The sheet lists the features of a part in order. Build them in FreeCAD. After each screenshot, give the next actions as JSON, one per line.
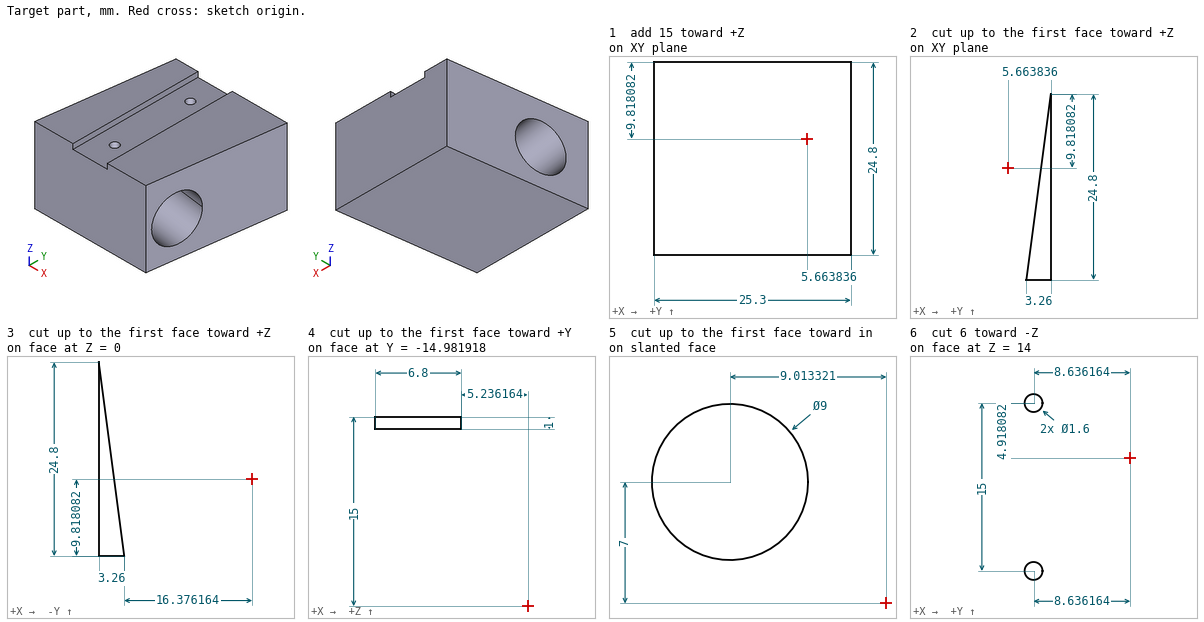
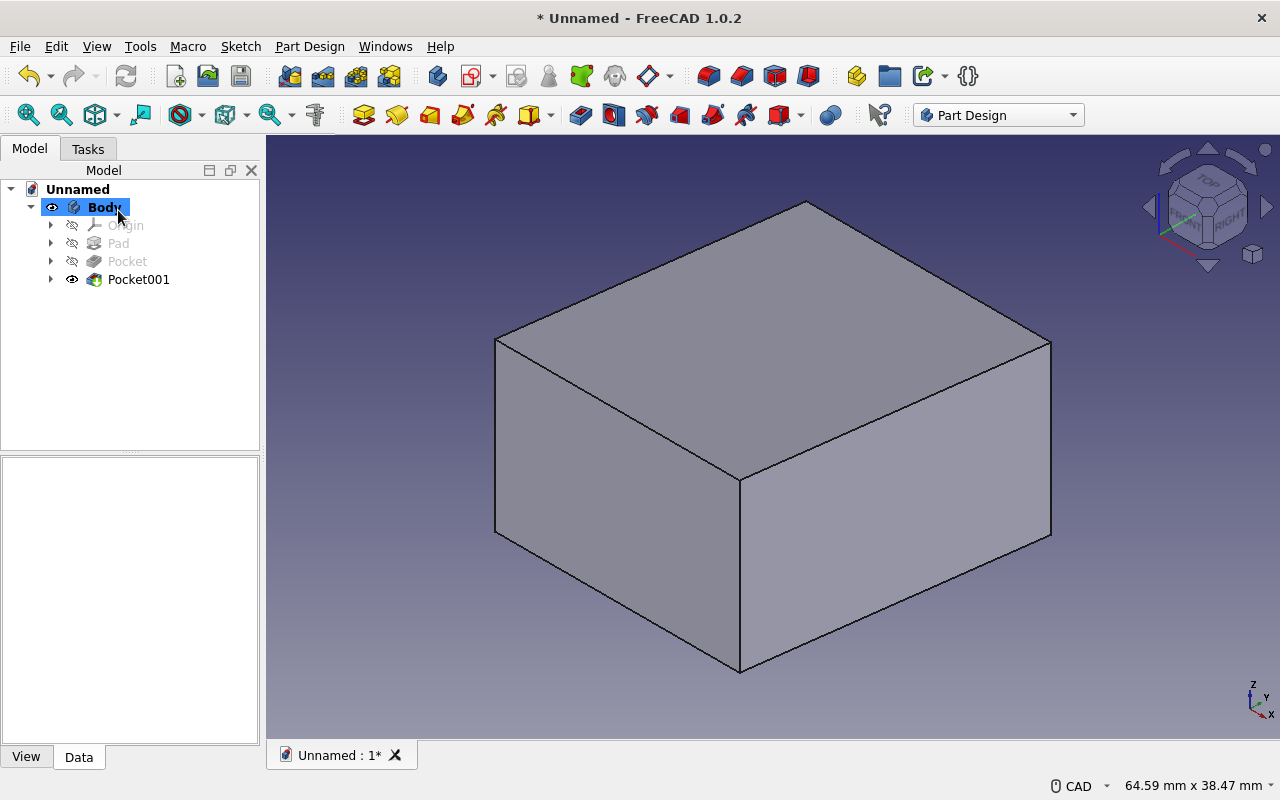
{"action": "left_click", "coordinate": [652, 525]}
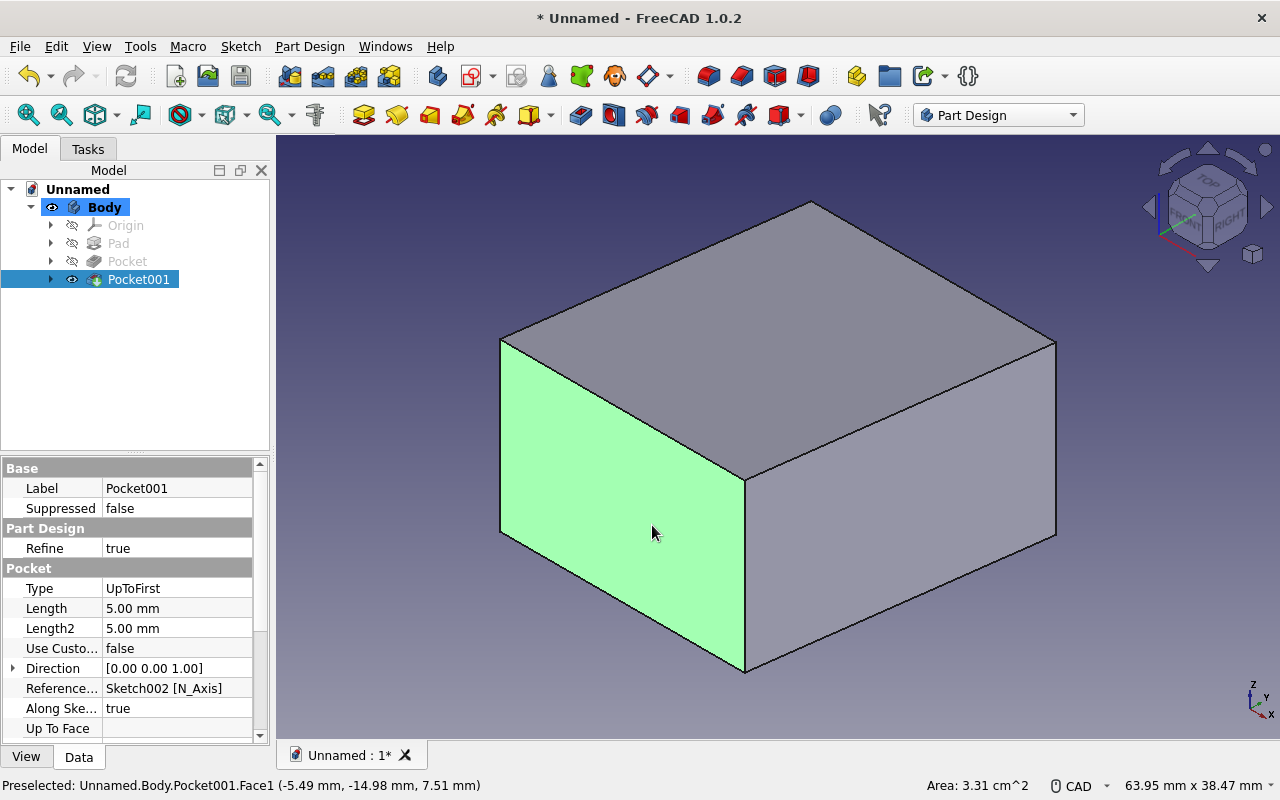
{"action": "left_click", "coordinate": [470, 76]}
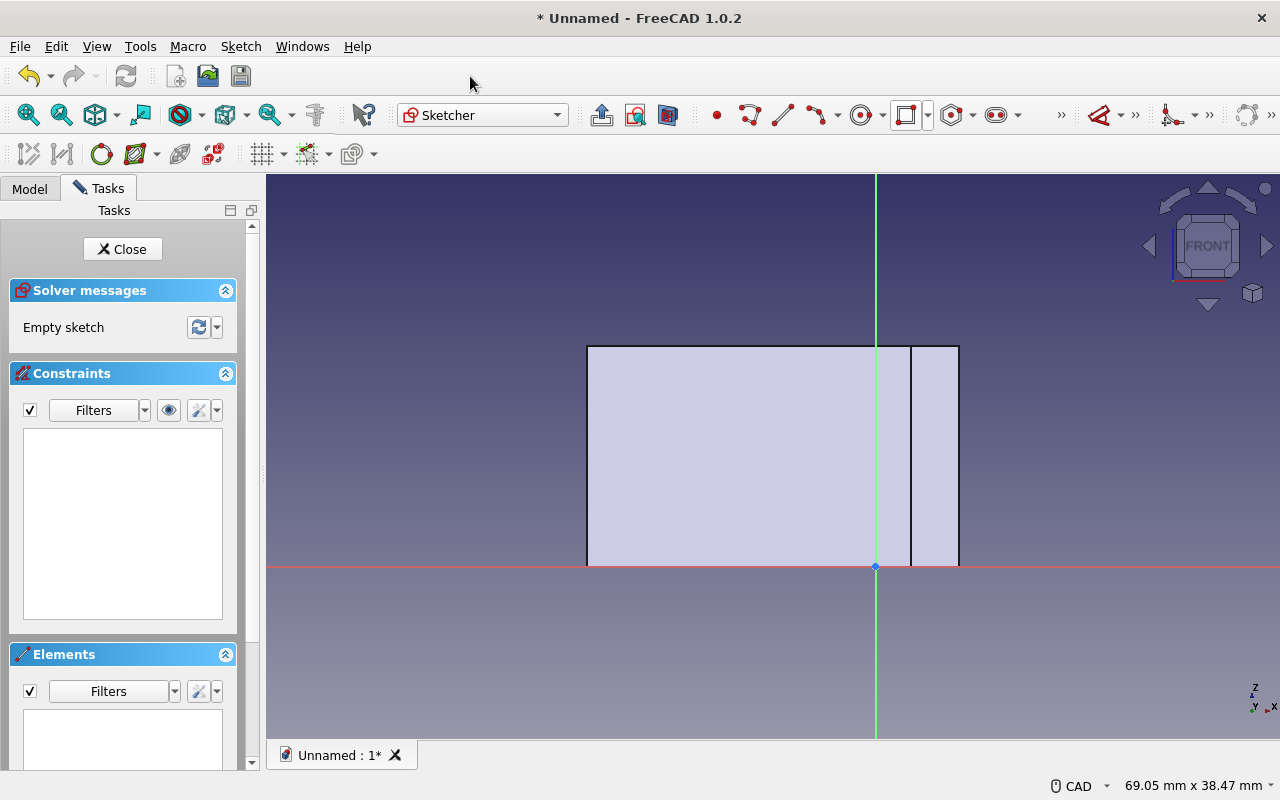
{"action": "scroll", "coordinate": [955, 456], "scroll_direction": "up", "scroll_amount": 2}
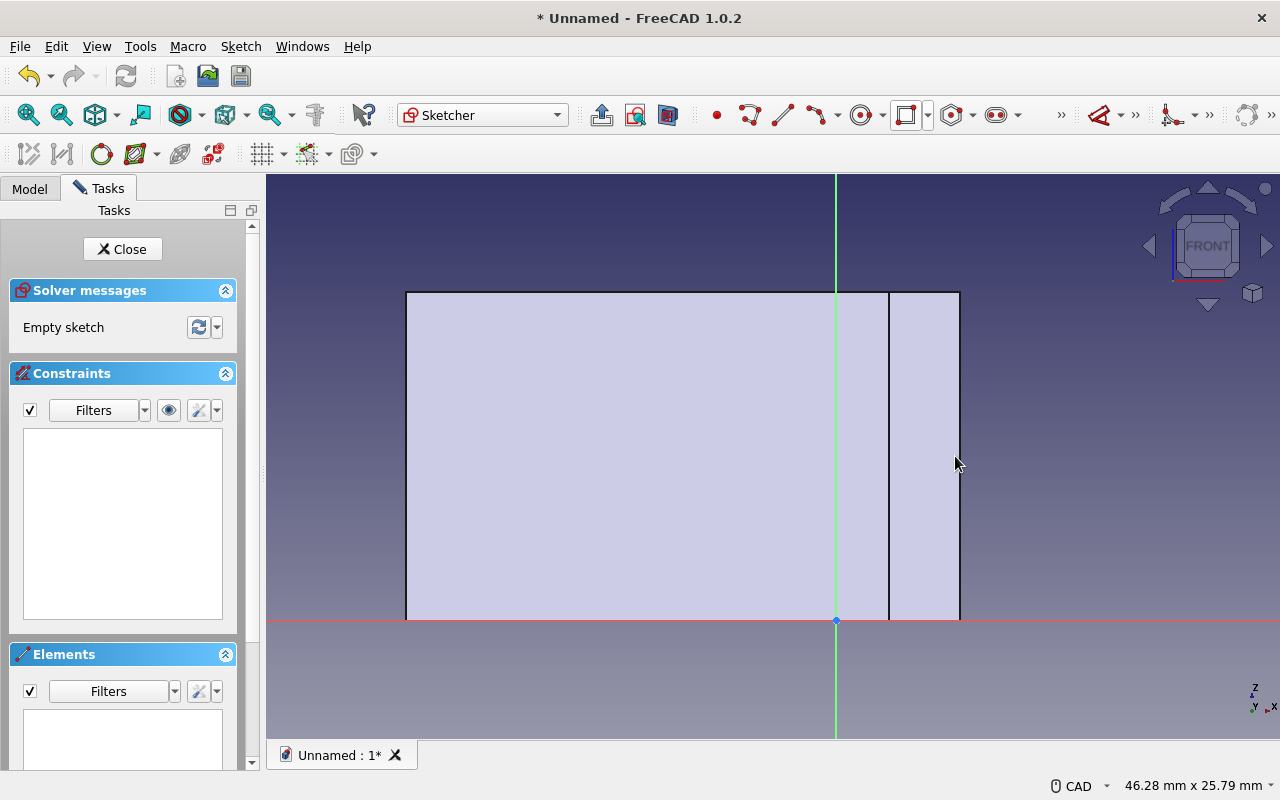
{"action": "left_click", "coordinate": [906, 116]}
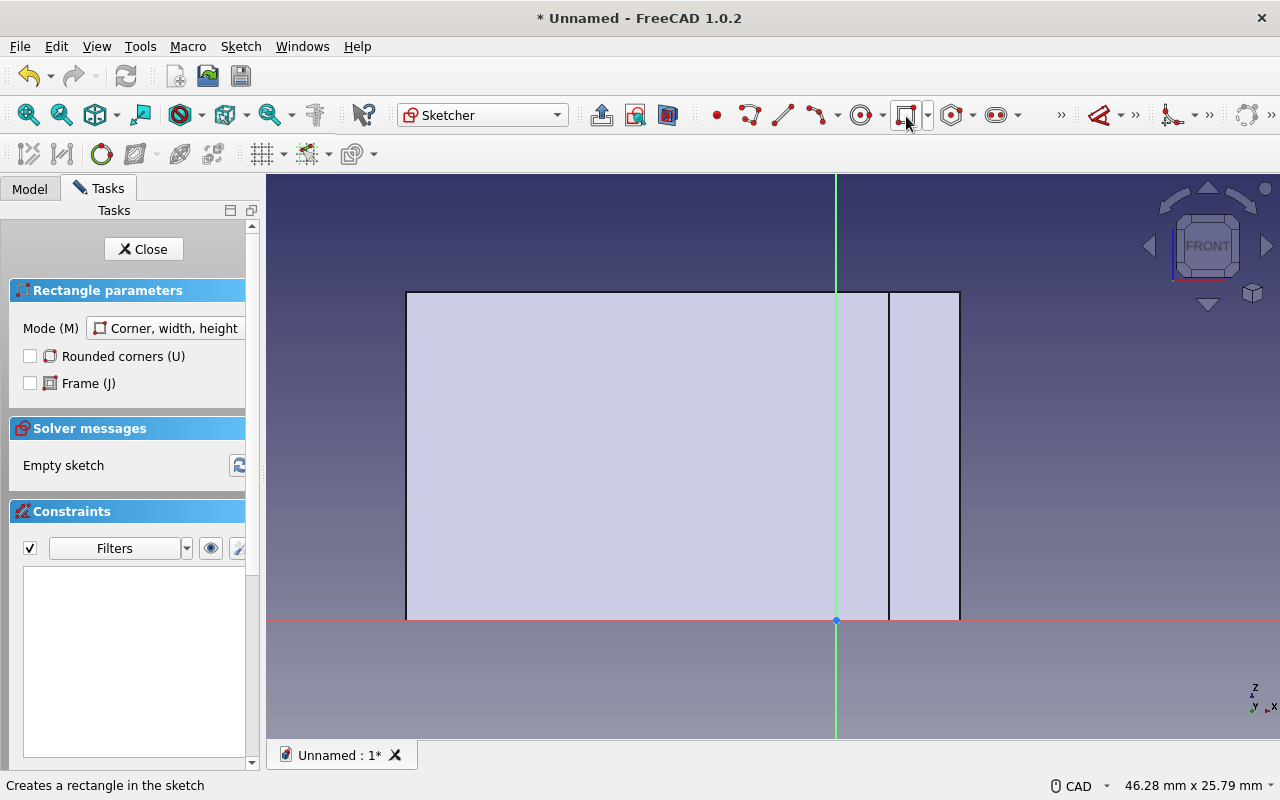
{"action": "left_click", "coordinate": [573, 292]}
{"action": "mouse_move", "coordinate": [721, 314]}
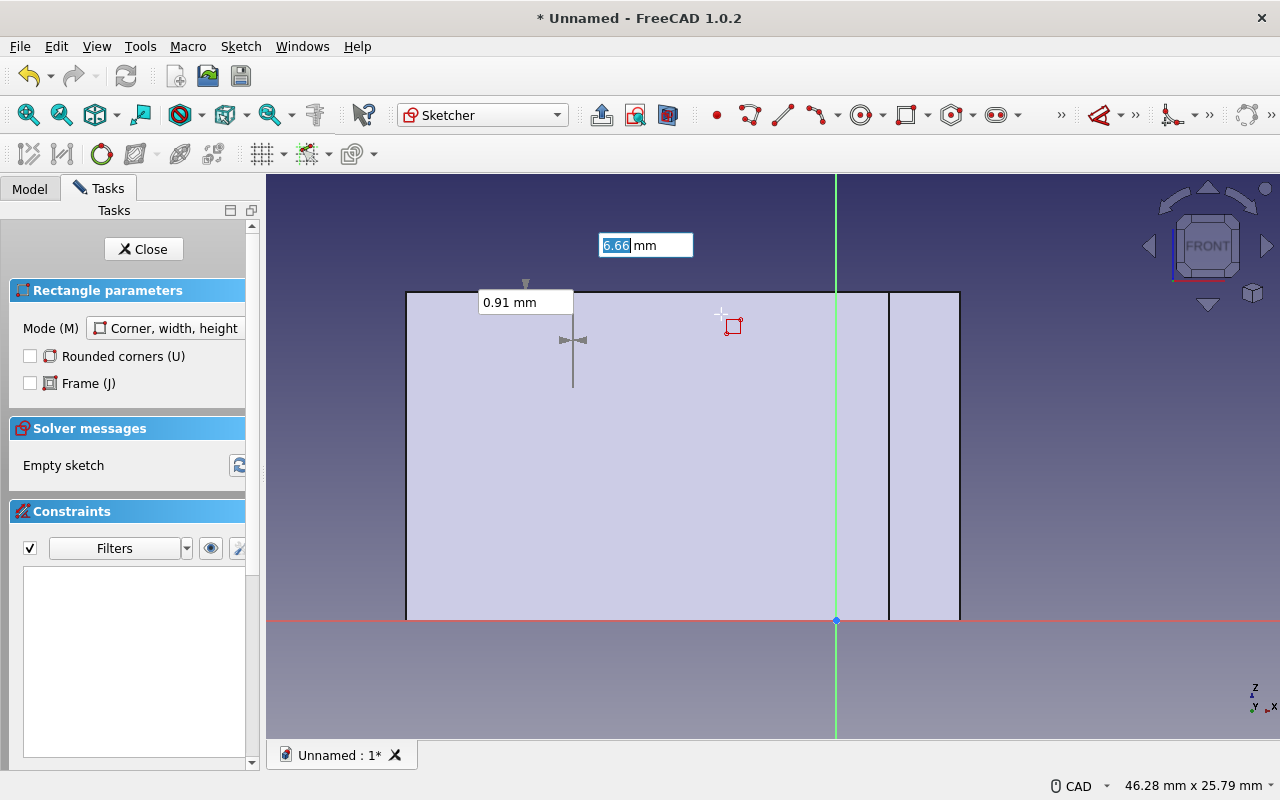
{"action": "type", "text": "6.8"}
{"action": "key", "text": "Tab"}
{"action": "type", "text": "1"}
{"action": "key", "text": "Return"}
{"action": "key", "text": "Escape"}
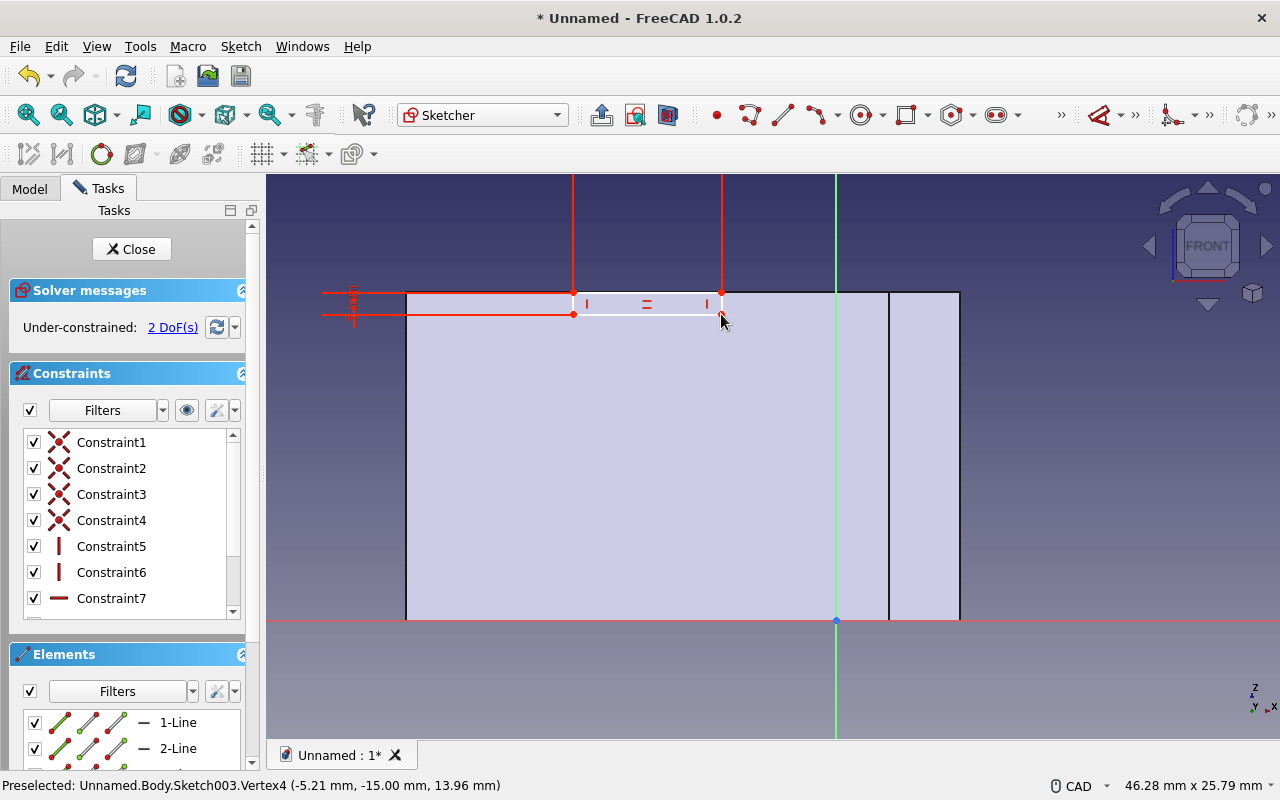
{"action": "left_click", "coordinate": [1098, 116]}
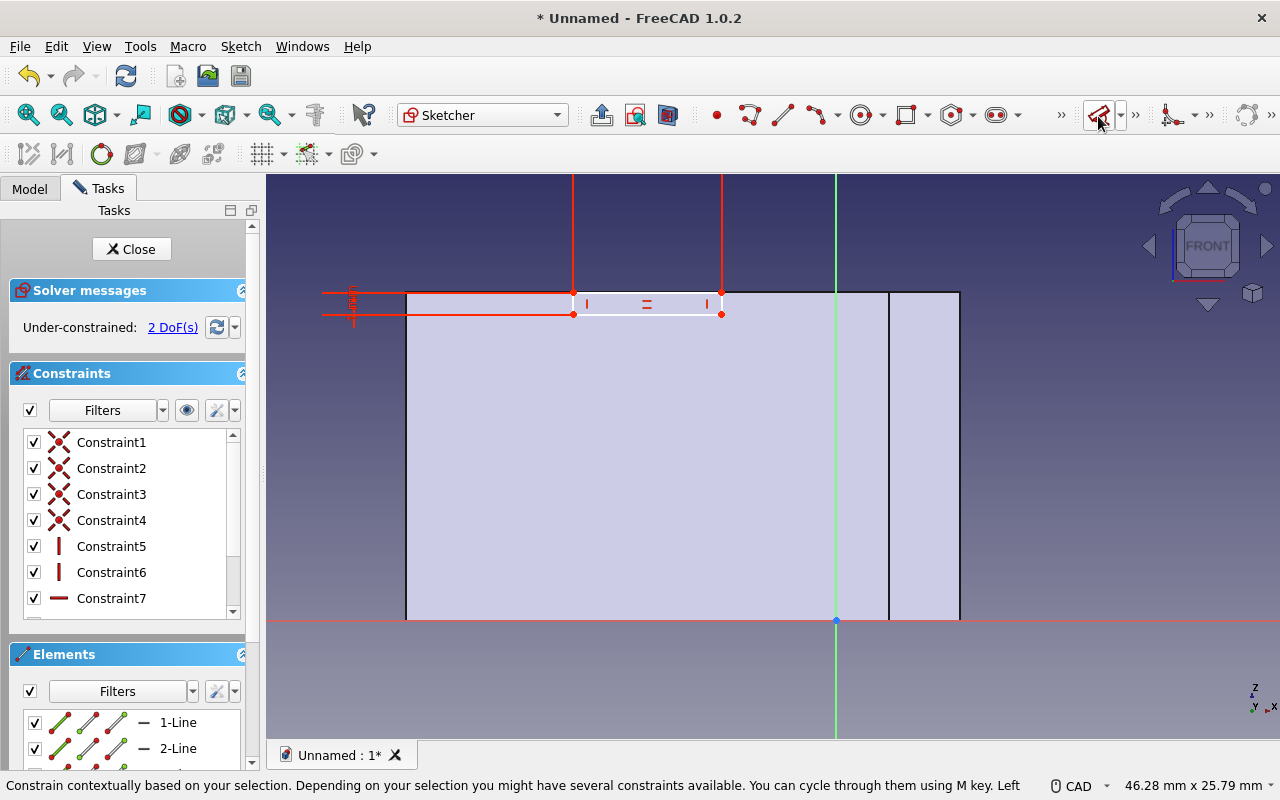
{"action": "left_click", "coordinate": [573, 293]}
{"action": "left_click", "coordinate": [870, 457]}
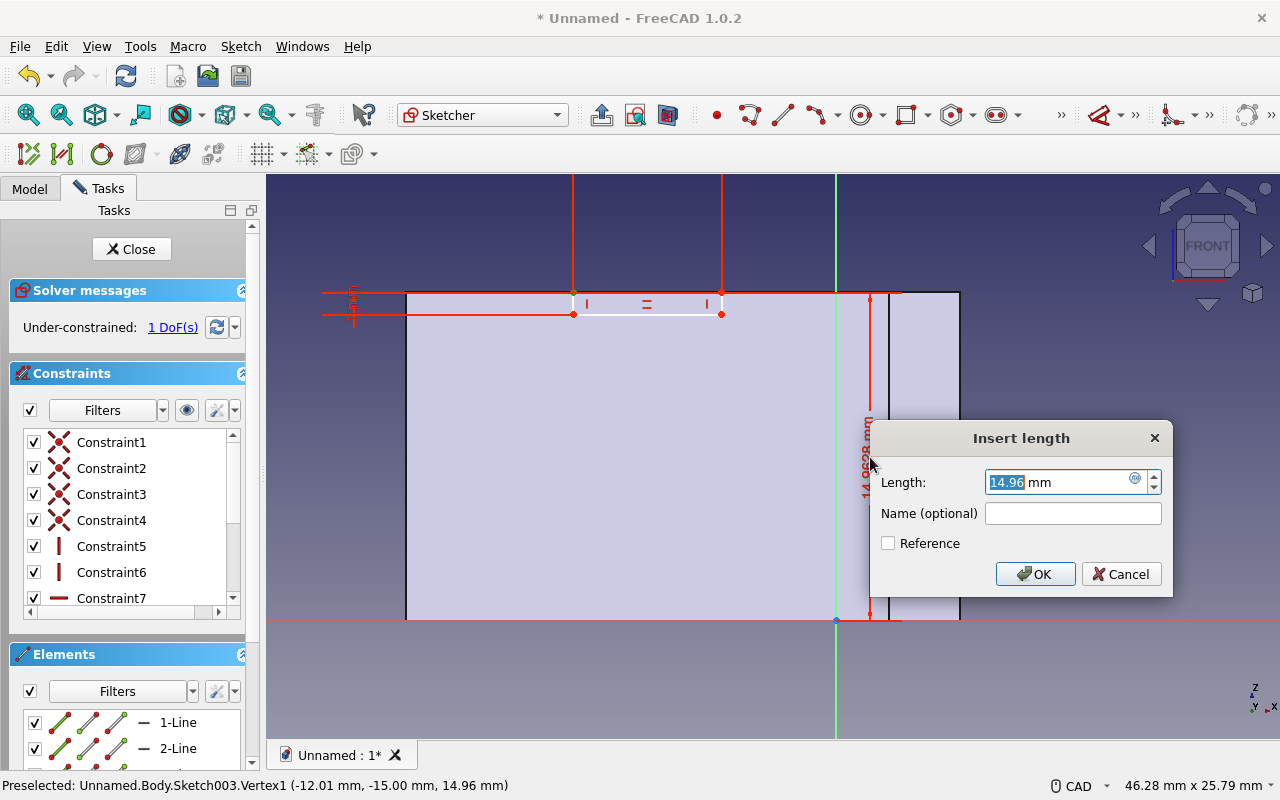
{"action": "type", "text": "15"}
{"action": "key", "text": "Return"}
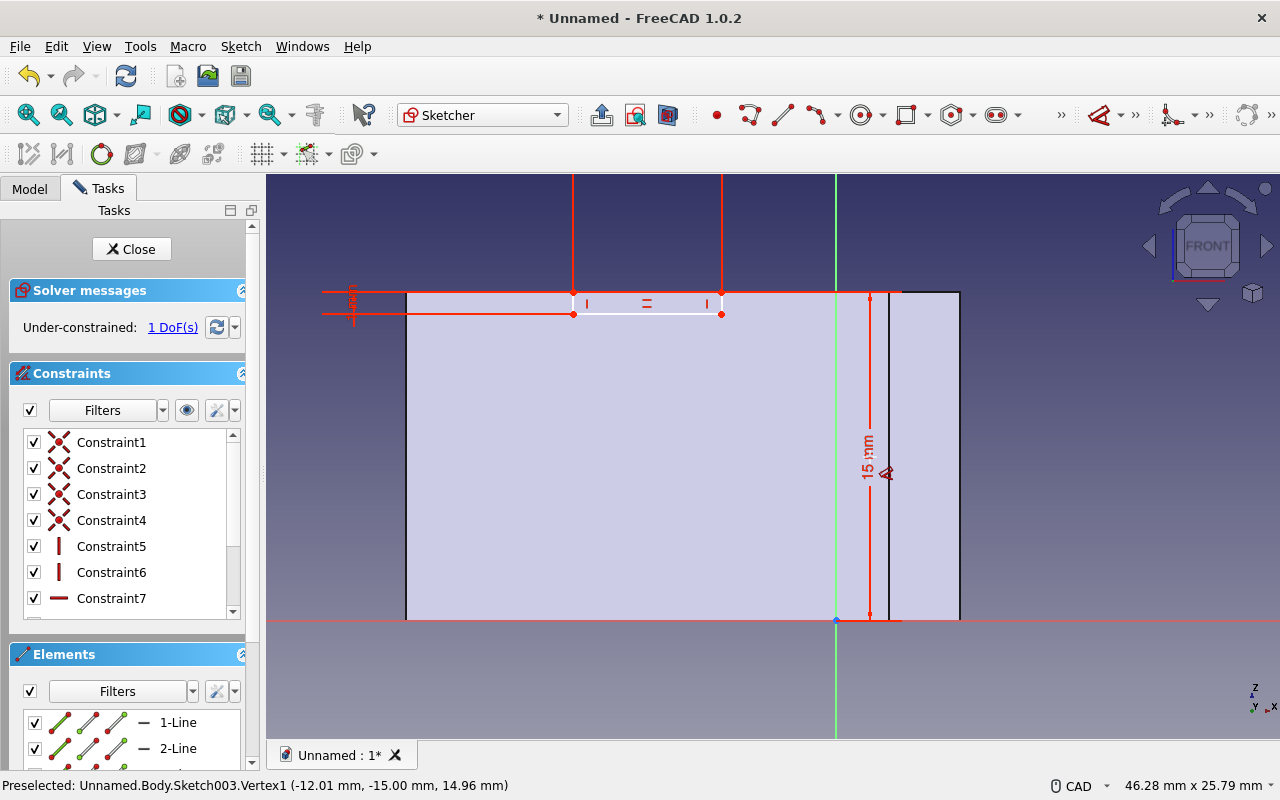
{"action": "left_click", "coordinate": [722, 314]}
{"action": "left_click", "coordinate": [779, 655]}